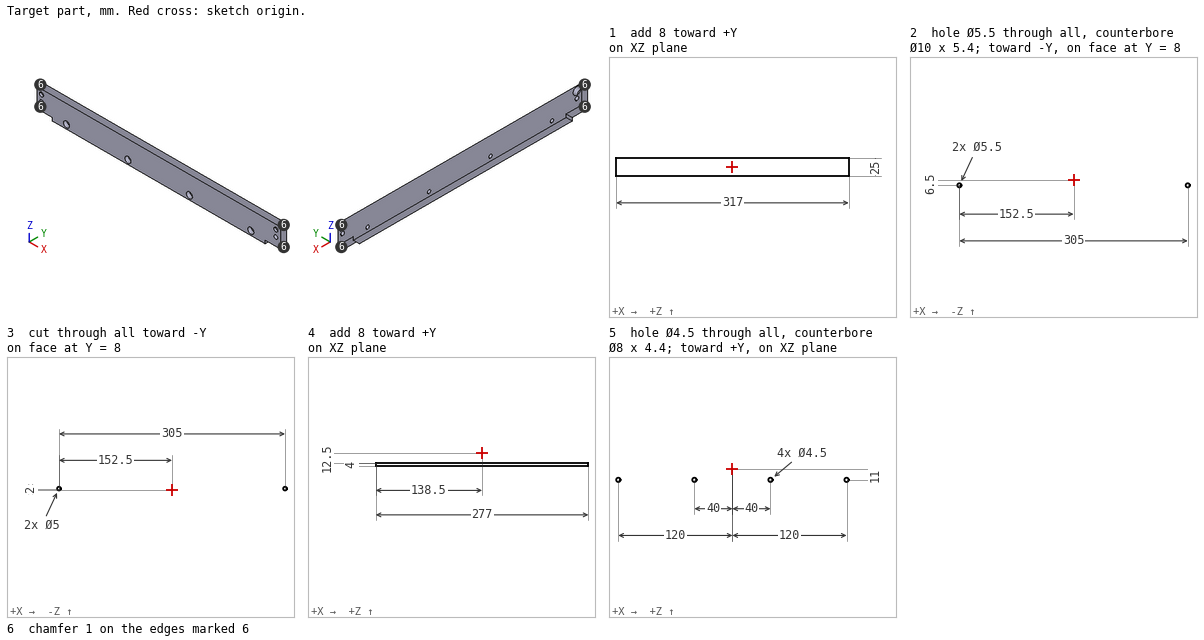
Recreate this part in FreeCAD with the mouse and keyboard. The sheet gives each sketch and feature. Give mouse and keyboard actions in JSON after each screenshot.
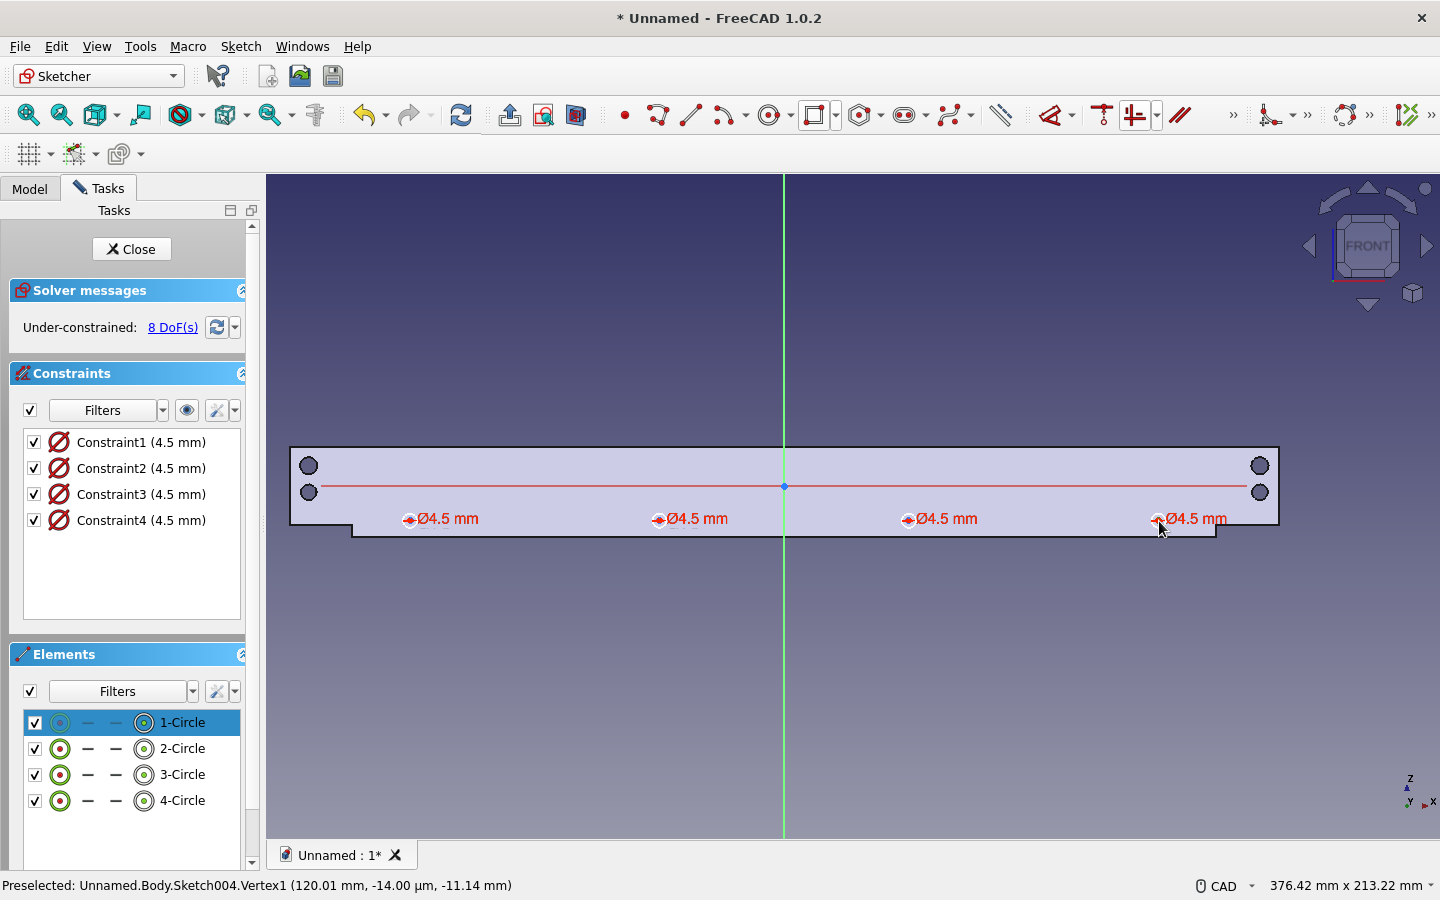
{"action": "left_click", "coordinate": [909, 521]}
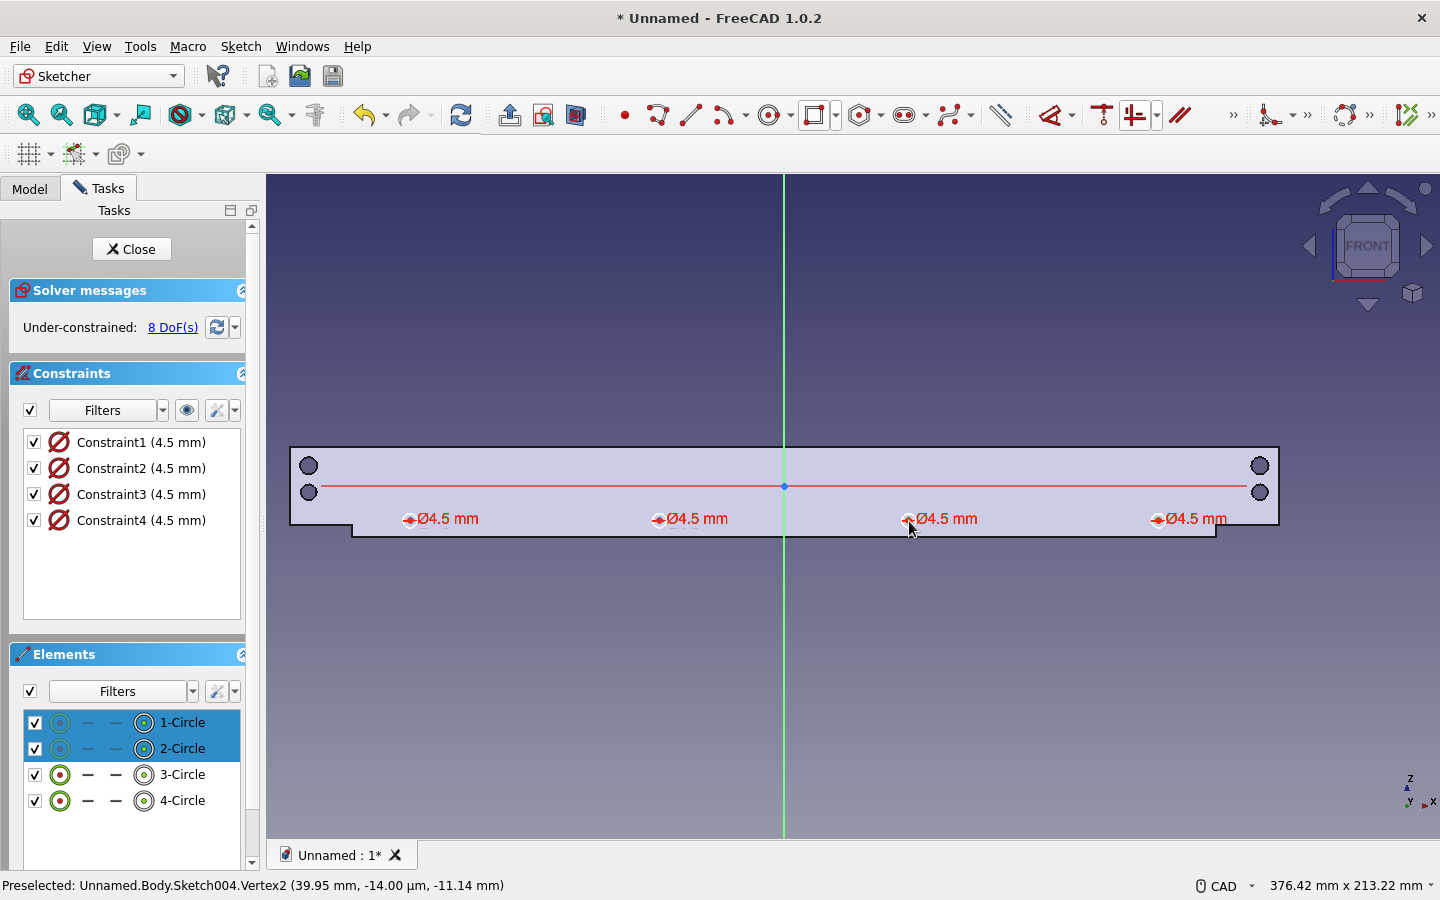
{"action": "left_click", "coordinate": [1156, 116]}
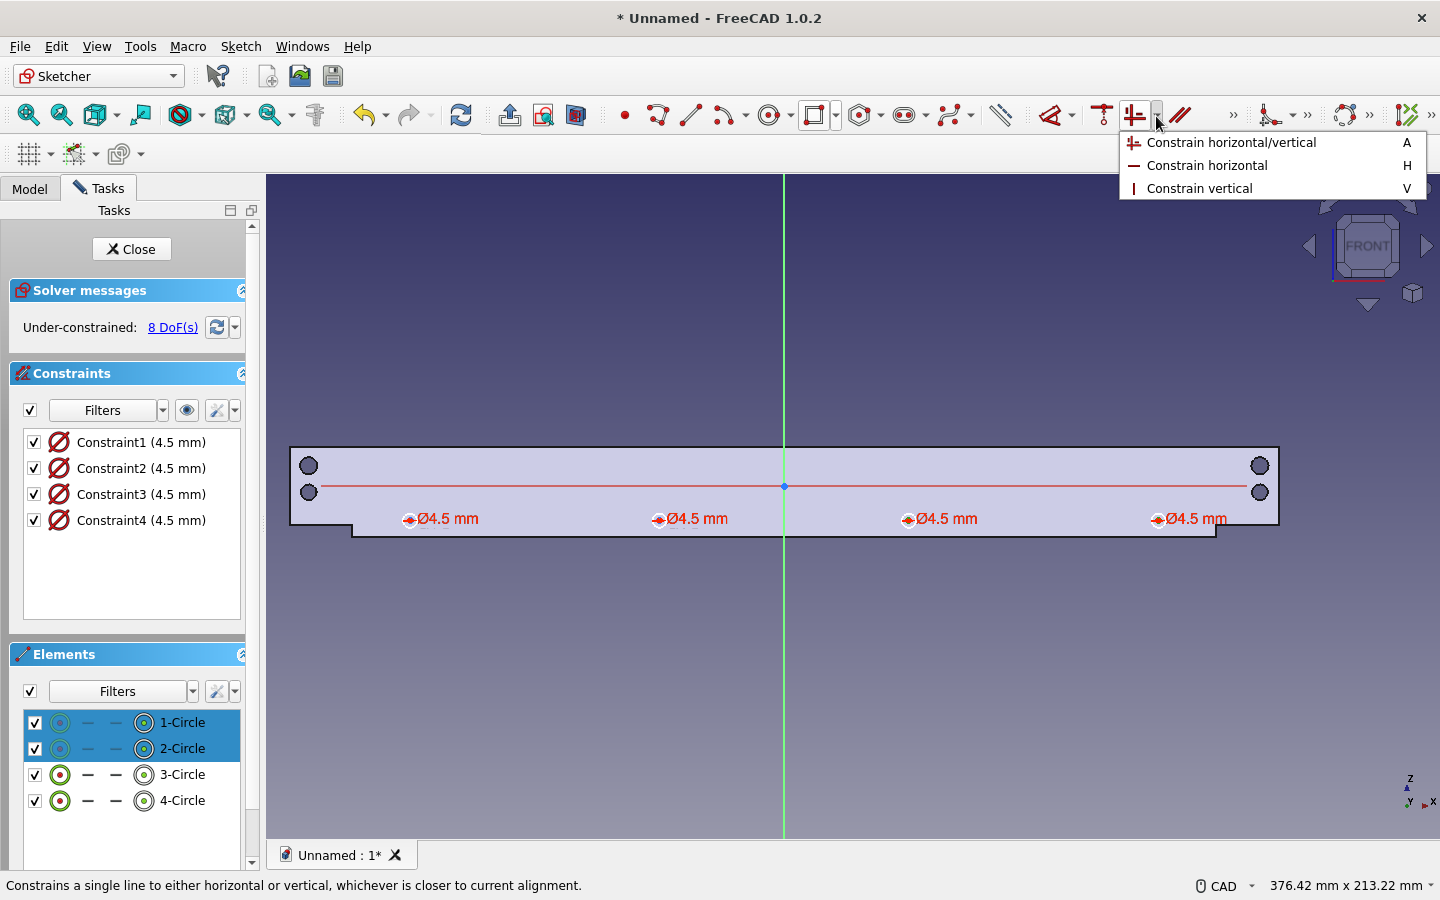
{"action": "left_click", "coordinate": [1273, 166]}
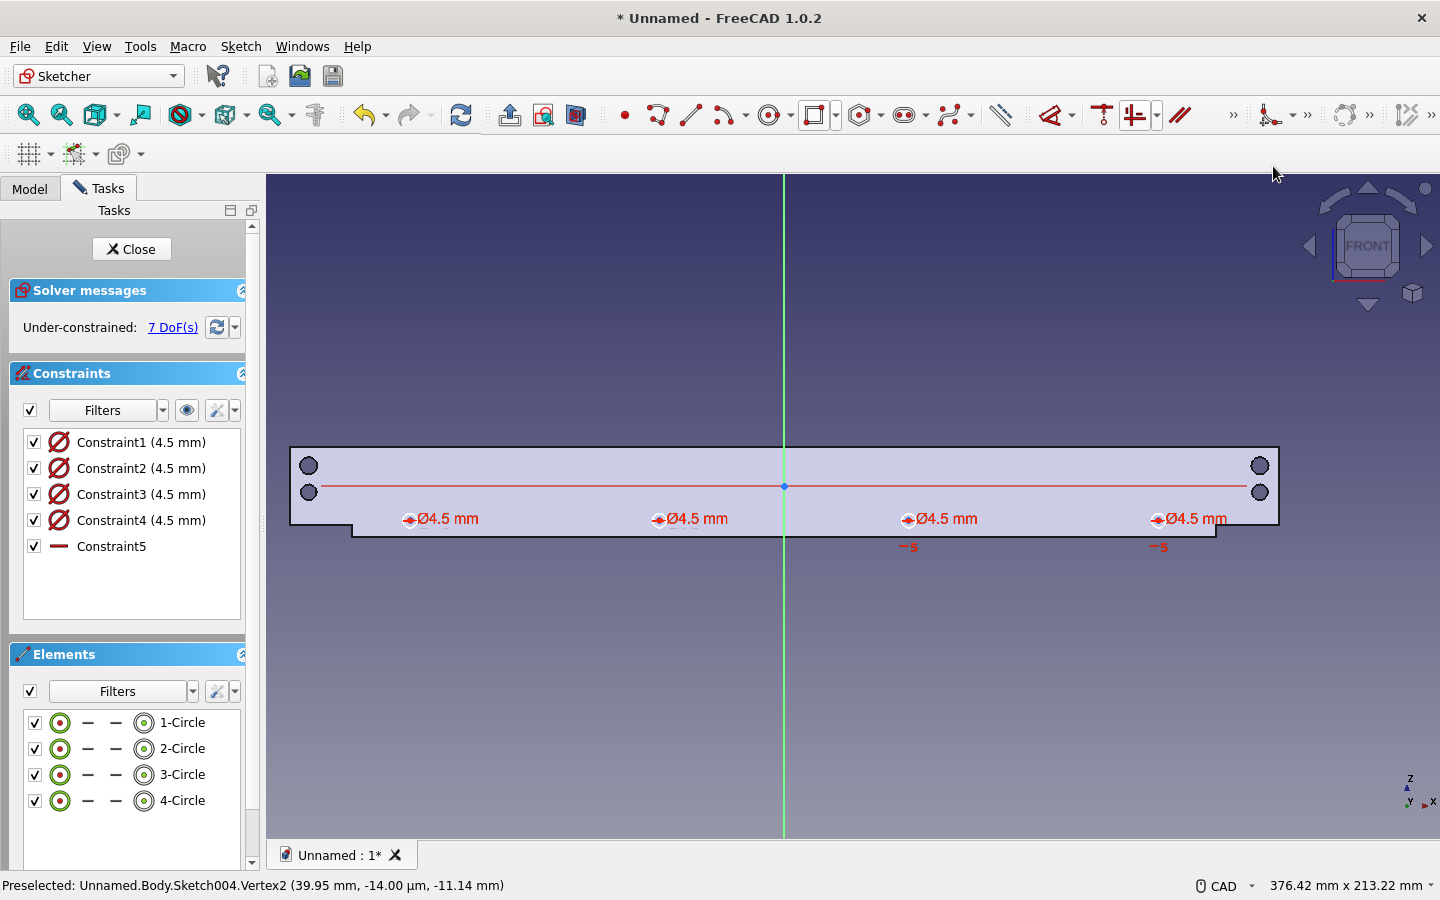
{"action": "left_click", "coordinate": [909, 521]}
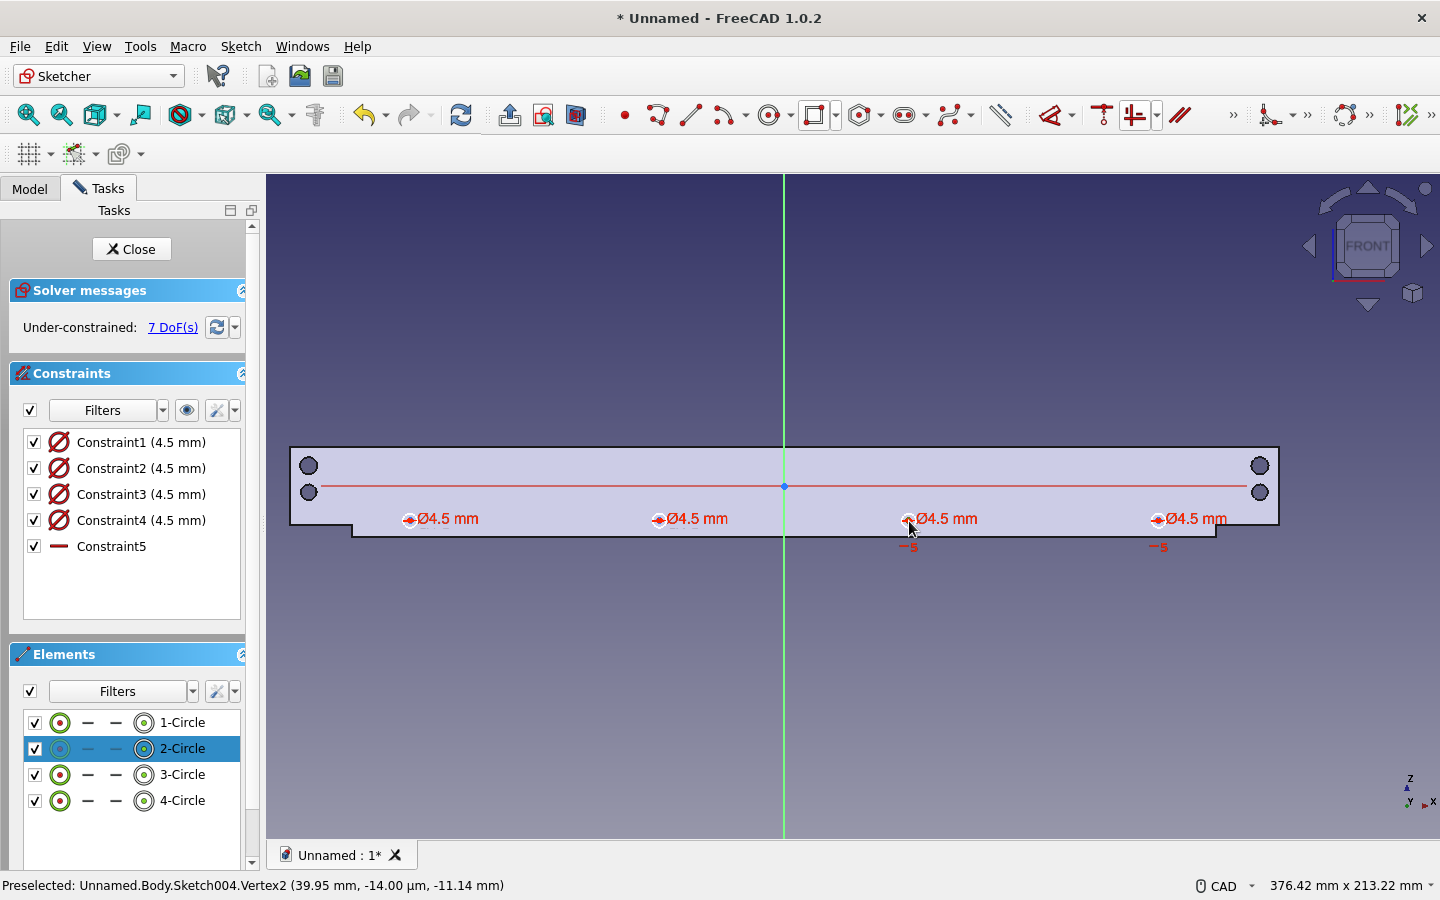
{"action": "left_click", "coordinate": [660, 521]}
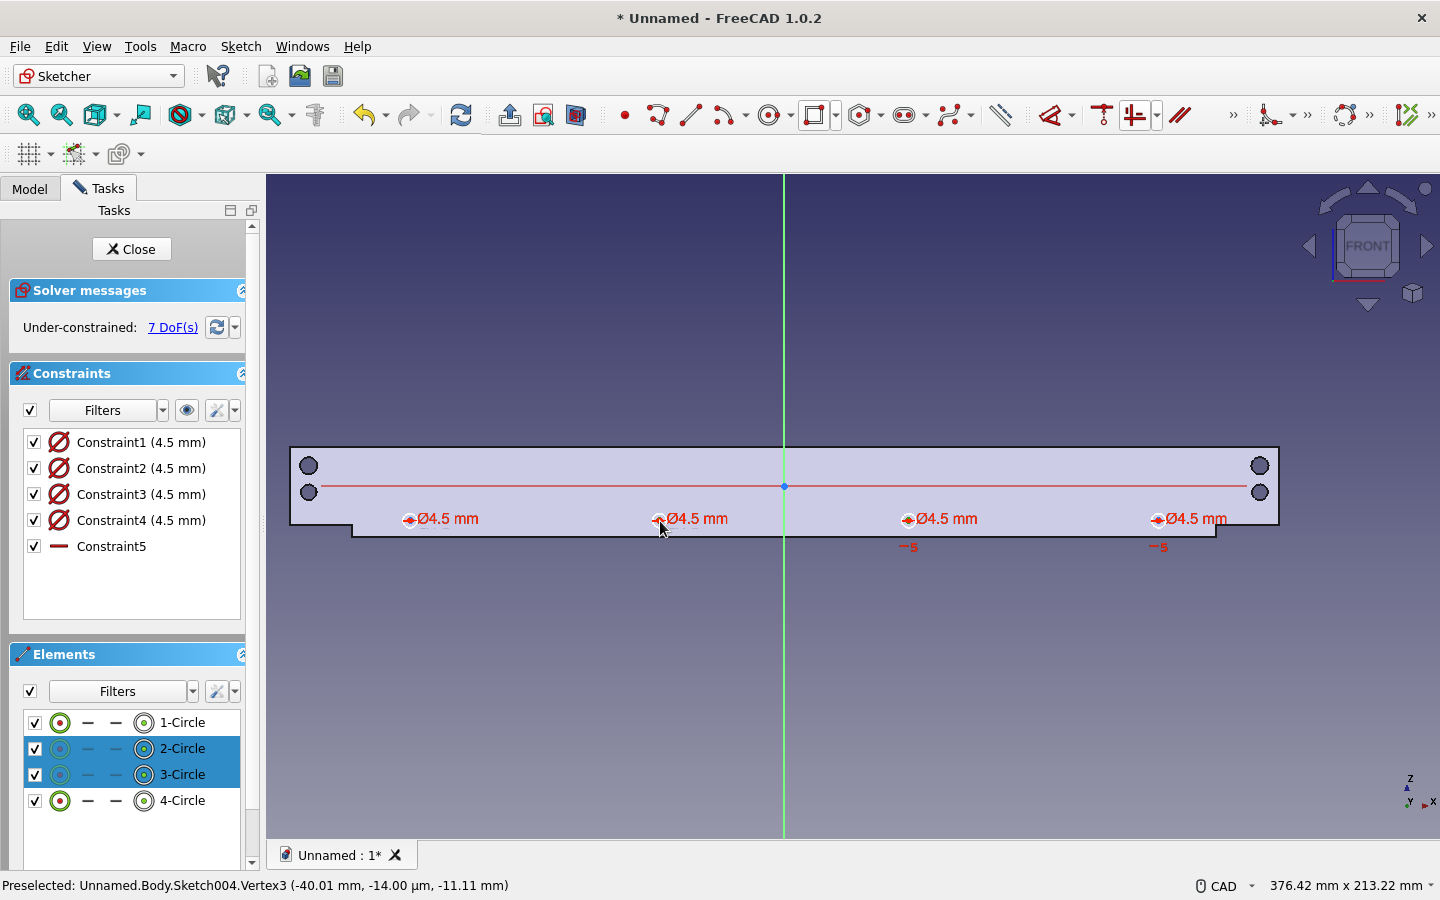
{"action": "key", "text": "h"}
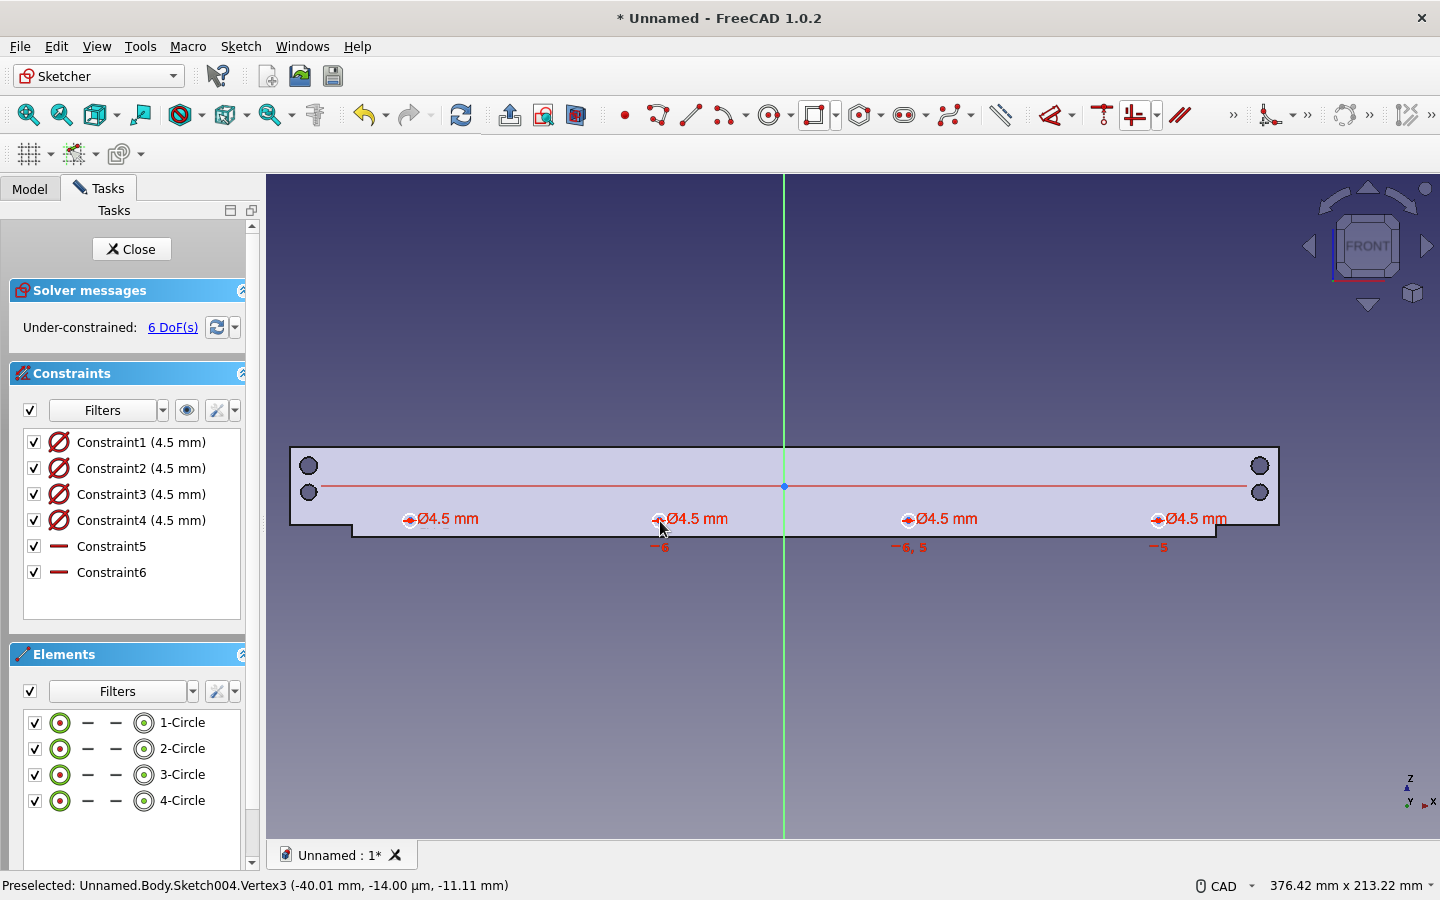
{"action": "left_click", "coordinate": [660, 521]}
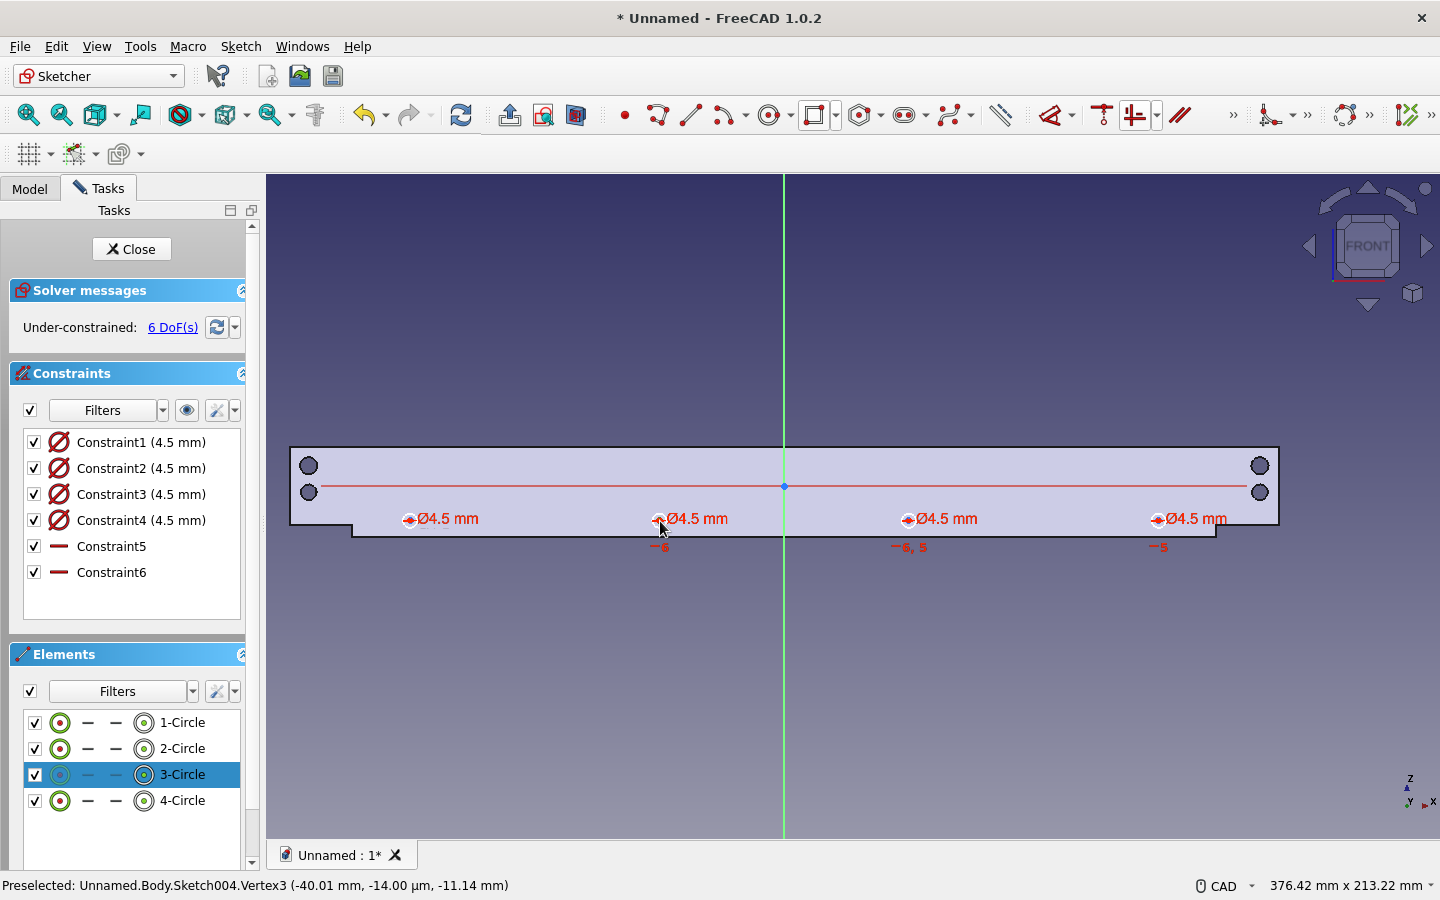
{"action": "left_click", "coordinate": [410, 521]}